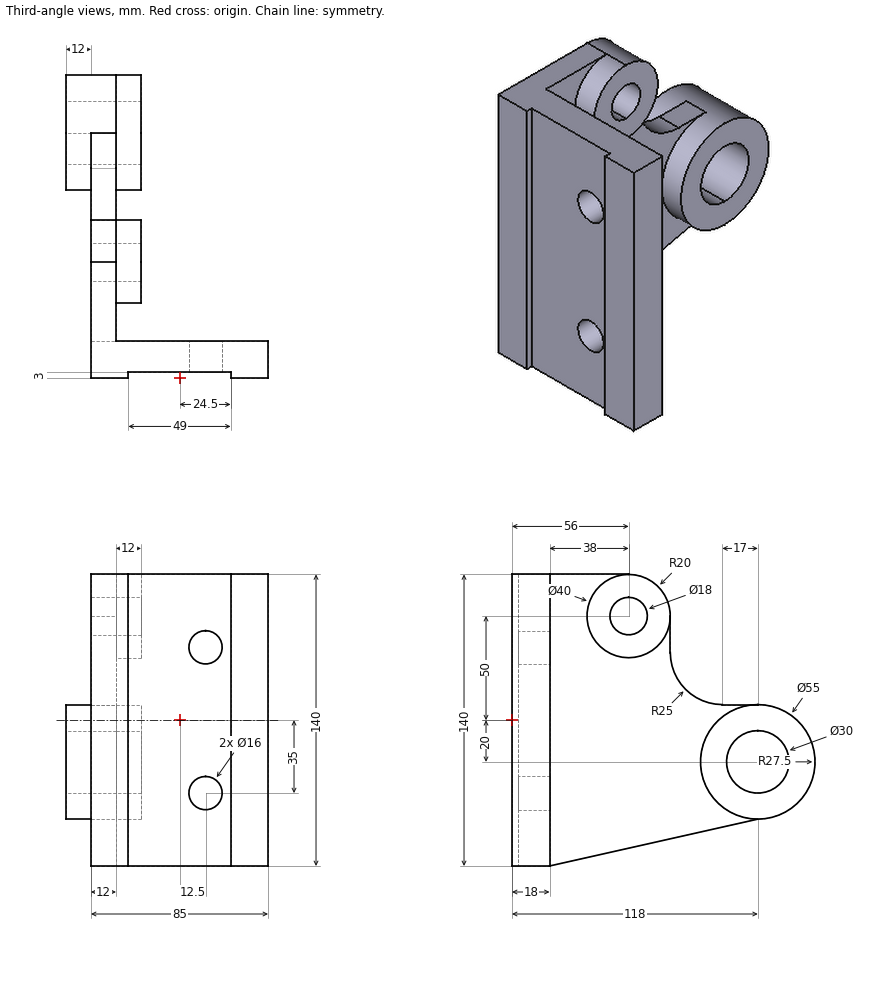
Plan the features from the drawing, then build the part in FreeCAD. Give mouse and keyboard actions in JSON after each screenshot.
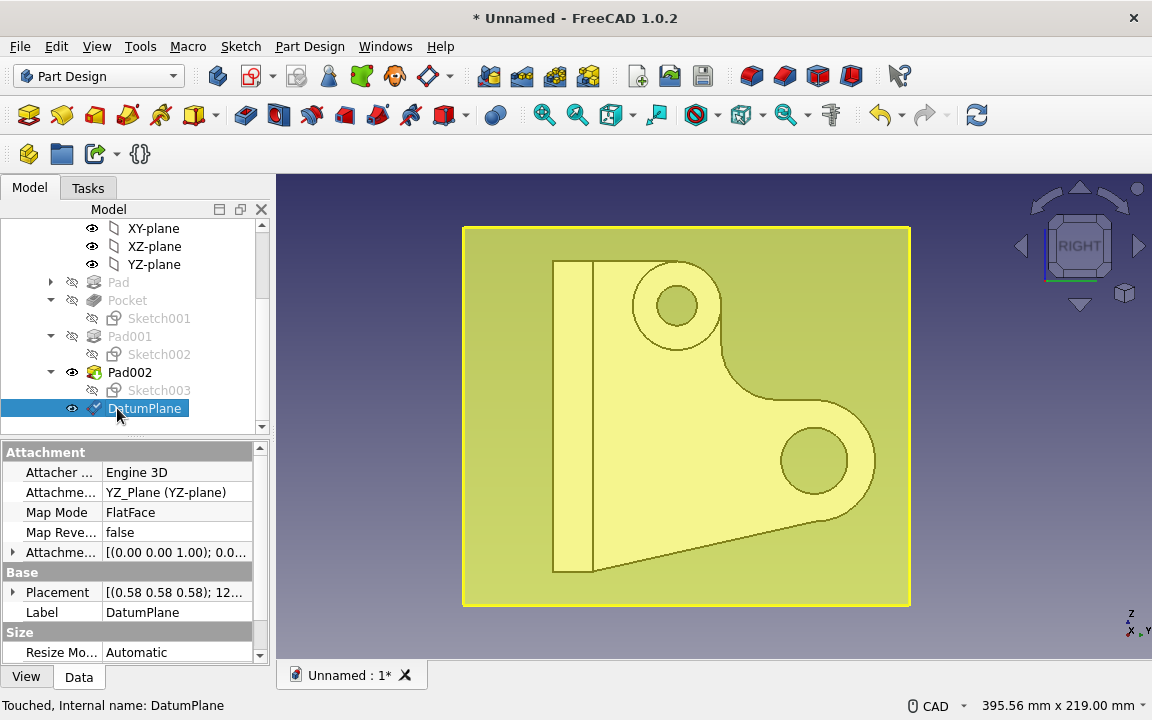
{"action": "left_click", "coordinate": [250, 76]}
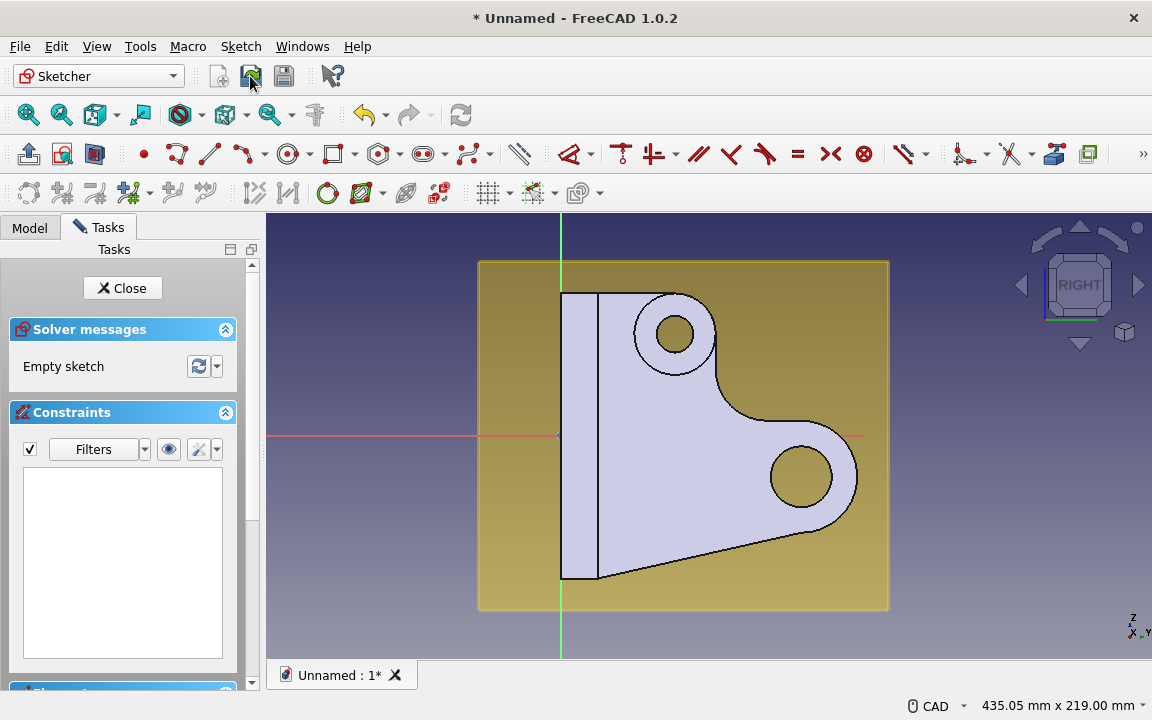
{"action": "key", "text": "q s"}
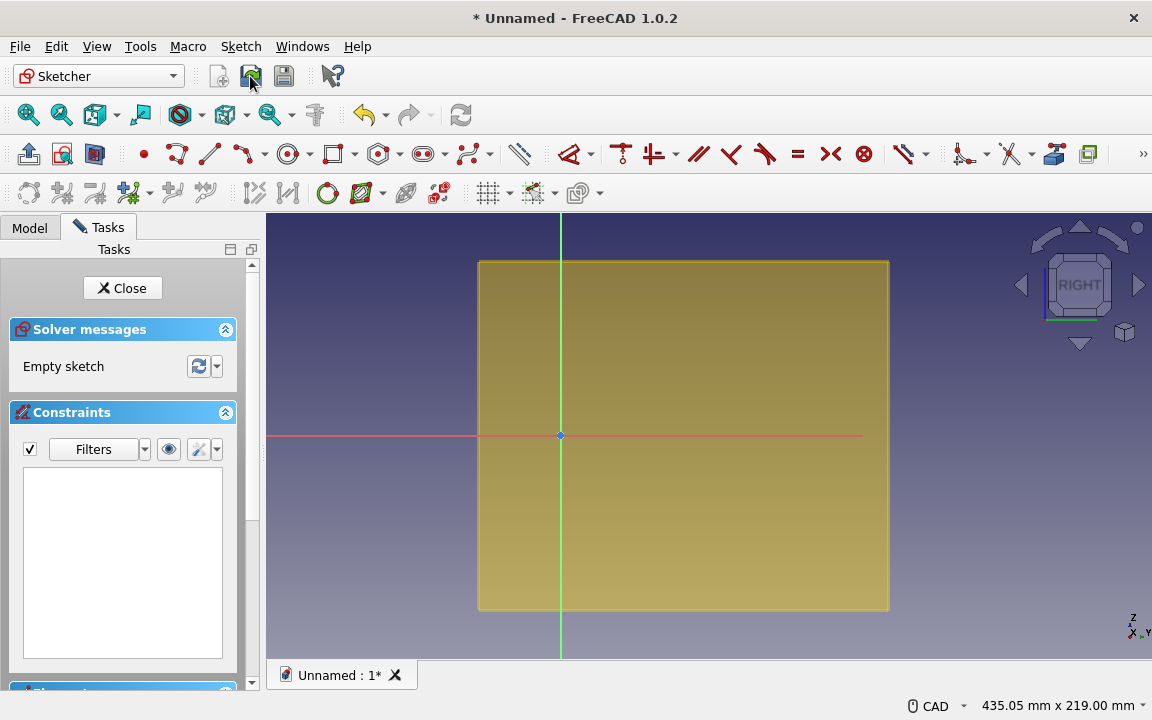
{"action": "scroll", "coordinate": [932, 510], "scroll_direction": "up", "scroll_amount": 4}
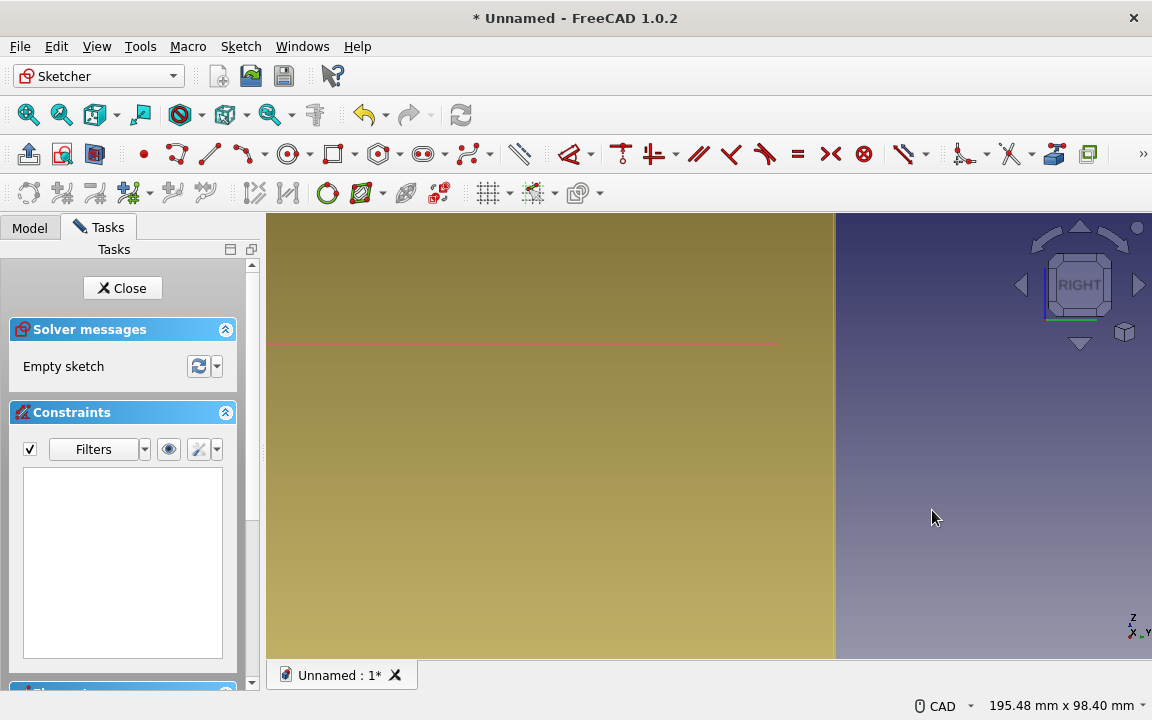
{"action": "key", "text": "g c"}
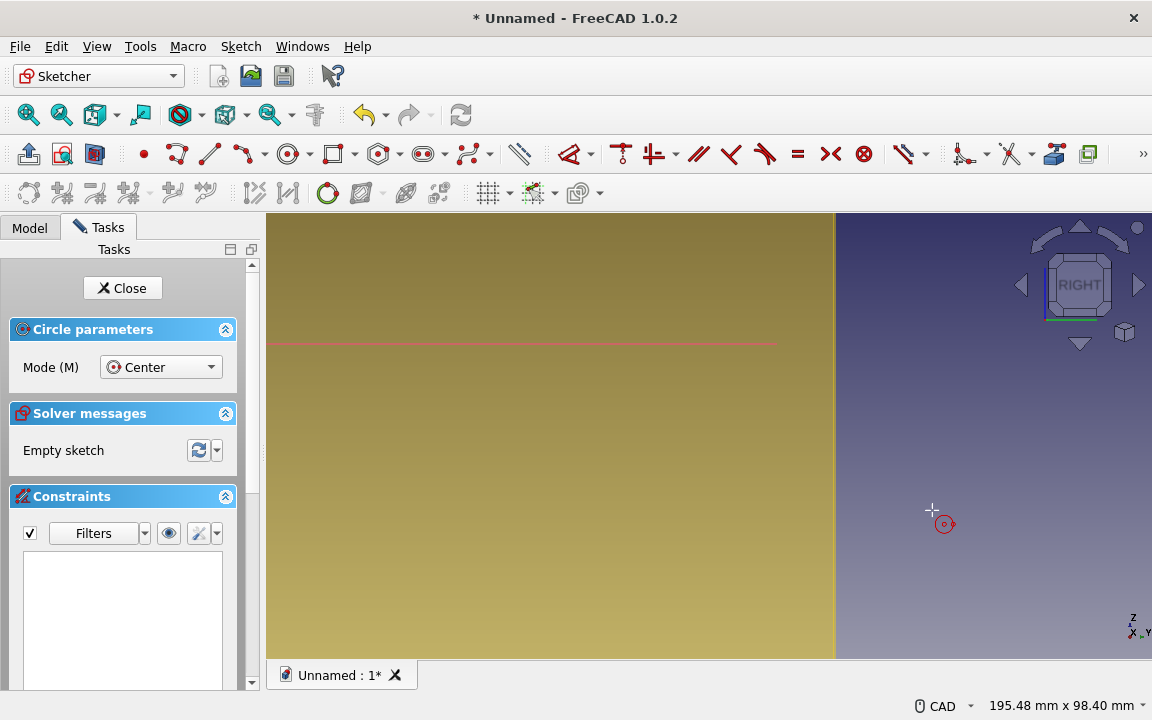
{"action": "left_click", "coordinate": [640, 435]}
{"action": "mouse_move", "coordinate": [728, 523]}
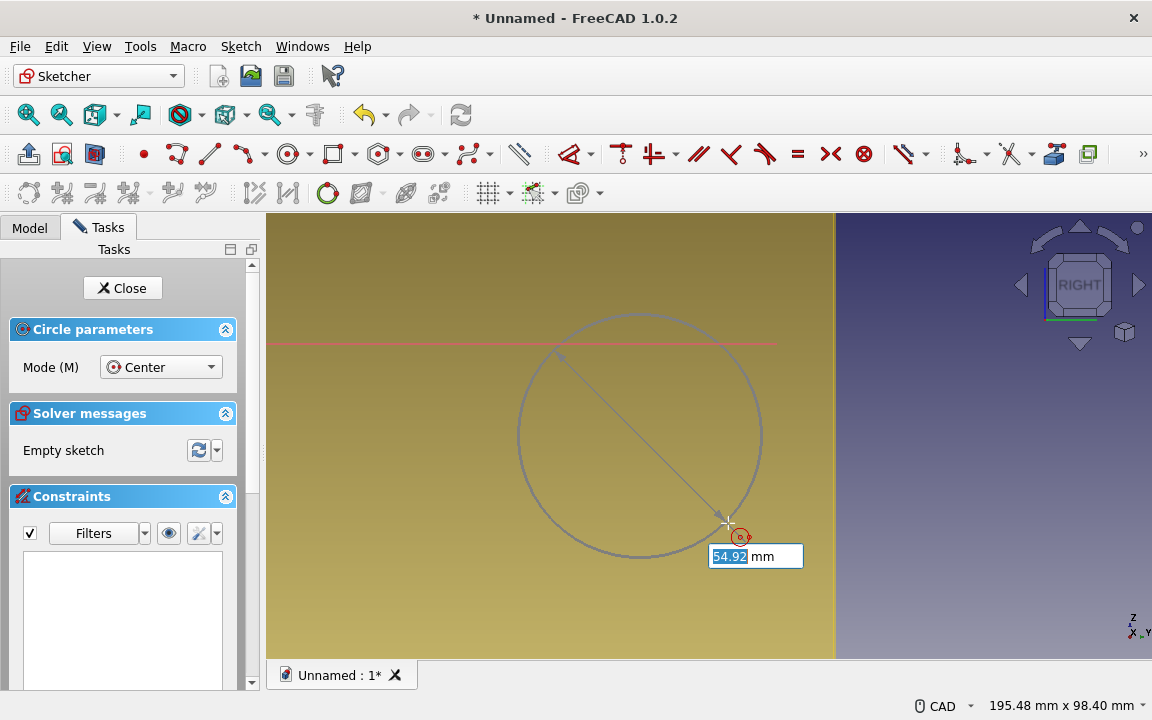
{"action": "type", "text": "55"}
{"action": "key", "text": "Return"}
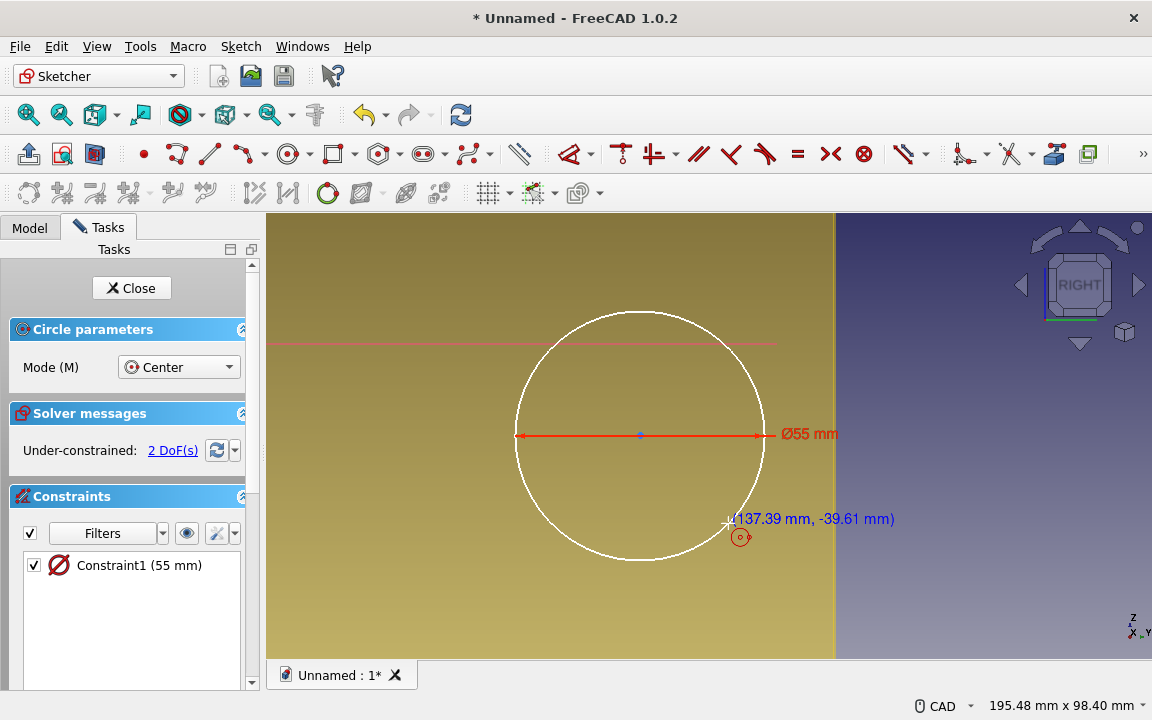
{"action": "left_click", "coordinate": [640, 436]}
{"action": "mouse_move", "coordinate": [688, 387]}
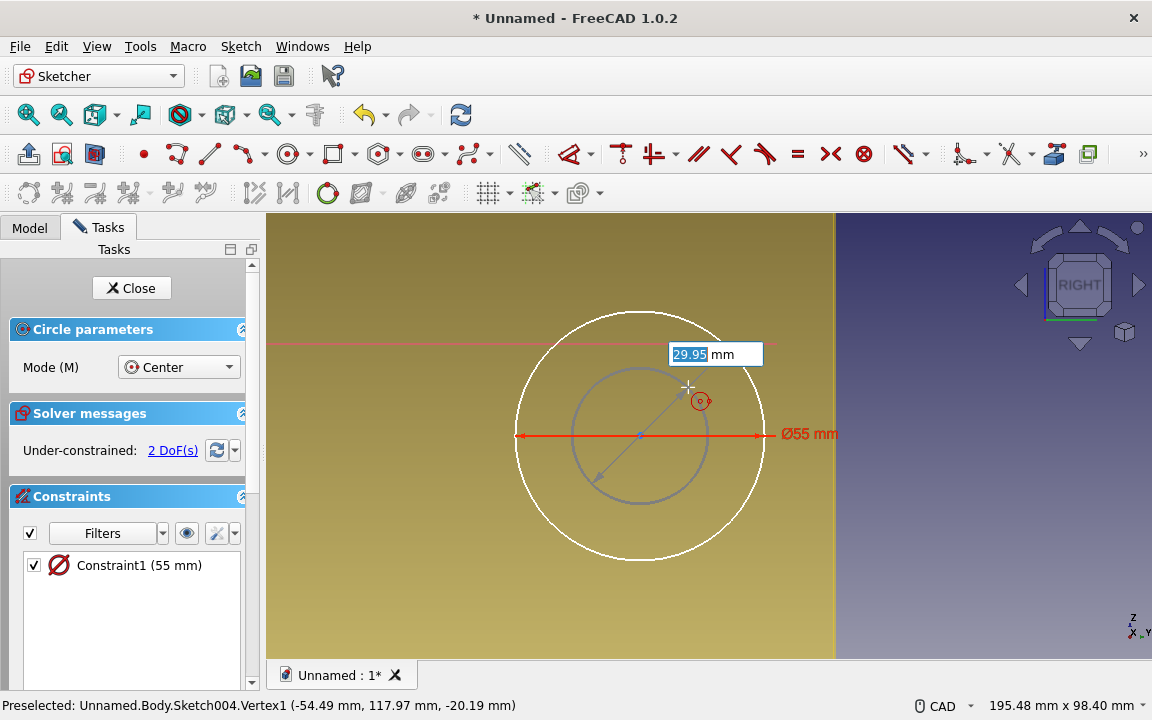
{"action": "type", "text": "30"}
{"action": "key", "text": "Return"}
{"action": "key", "text": "Escape"}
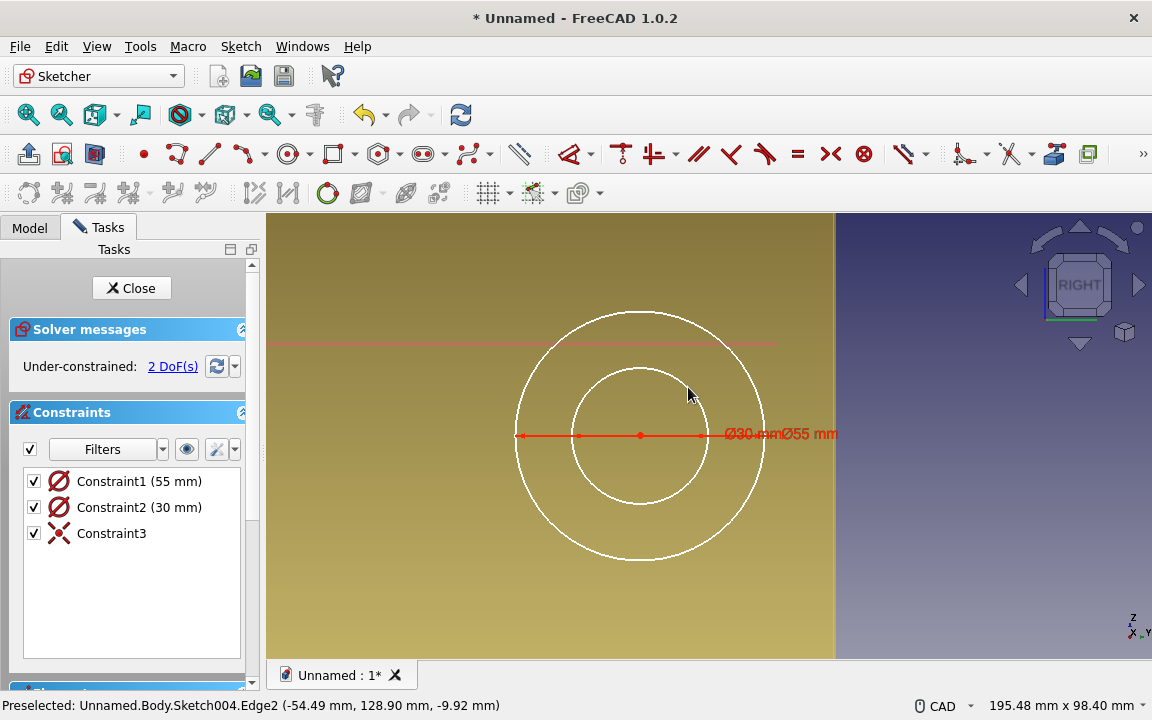
{"action": "left_click", "coordinate": [568, 154]}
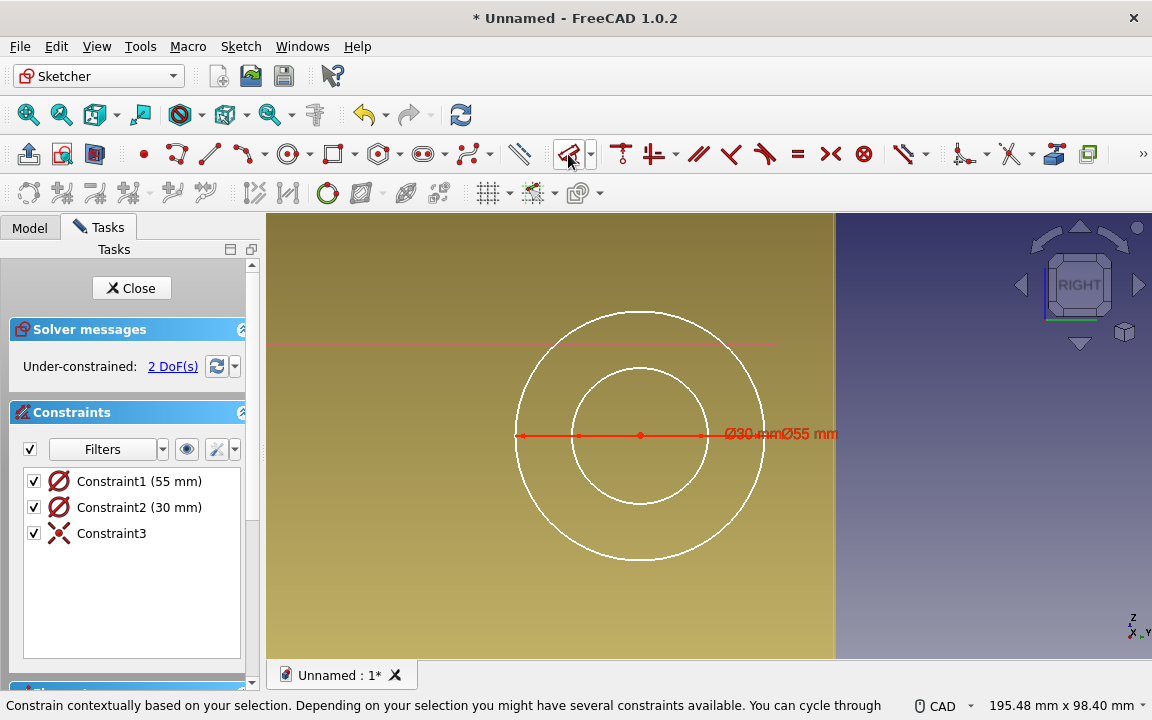
{"action": "left_click", "coordinate": [640, 436]}
{"action": "left_click", "coordinate": [674, 411]}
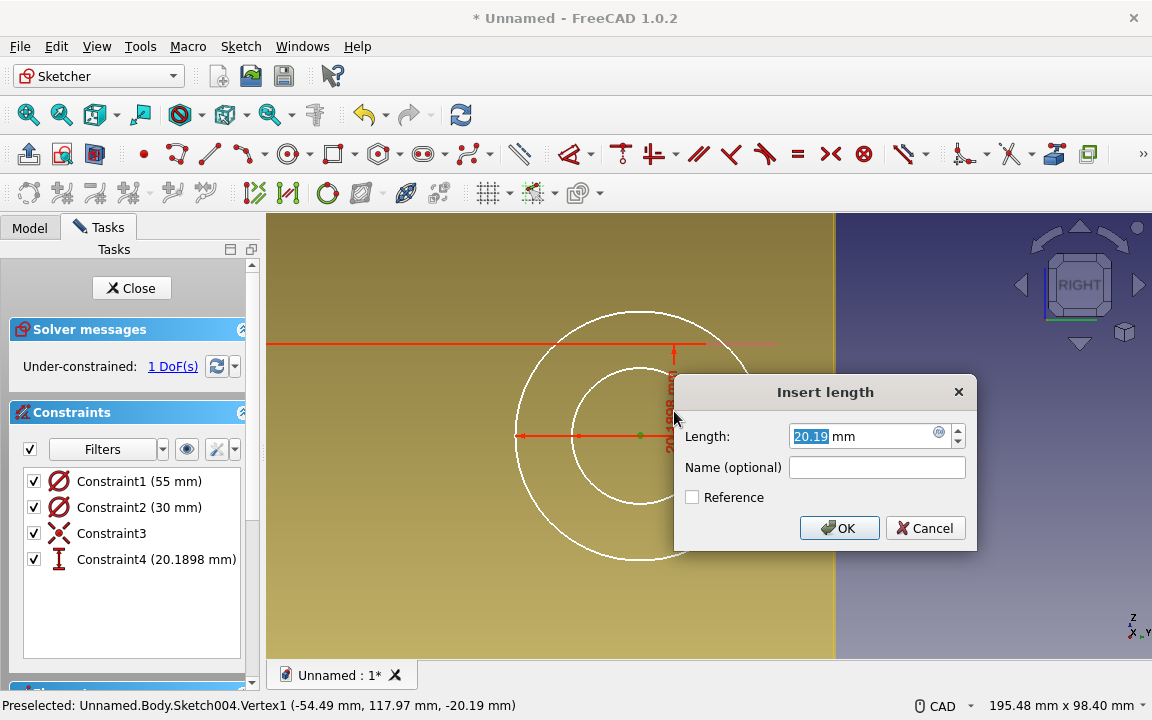
{"action": "type", "text": "20"}
{"action": "key", "text": "Return"}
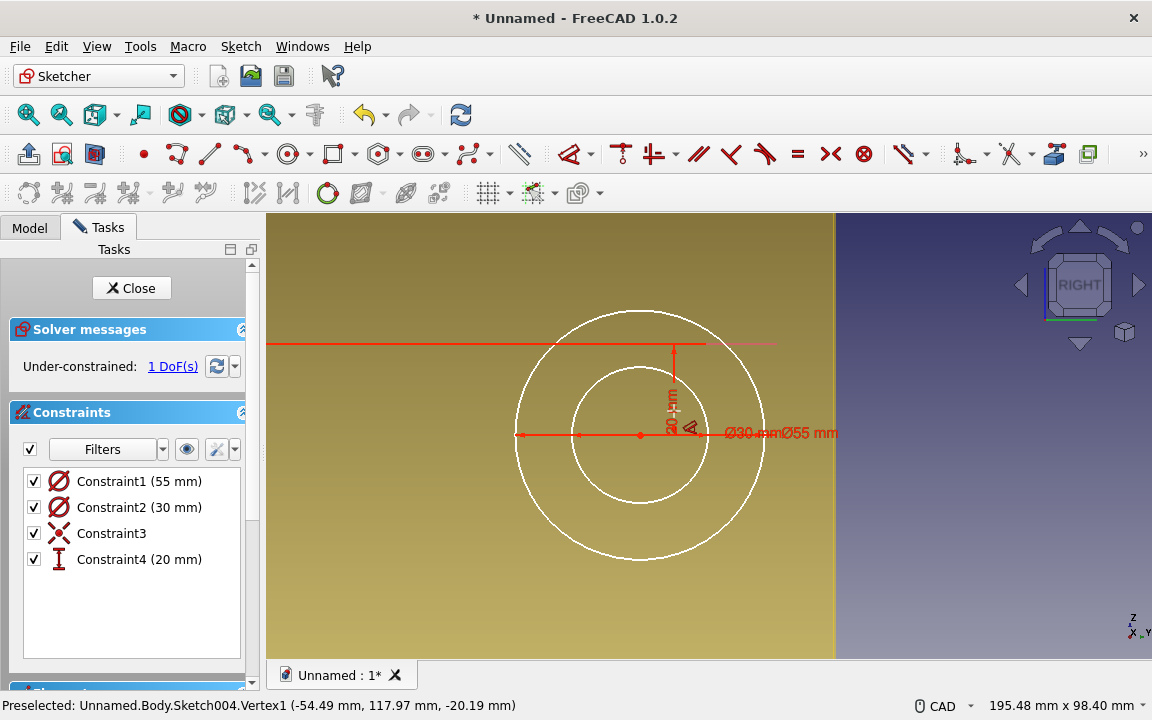
{"action": "left_click", "coordinate": [640, 435]}
{"action": "left_click", "coordinate": [467, 310]}